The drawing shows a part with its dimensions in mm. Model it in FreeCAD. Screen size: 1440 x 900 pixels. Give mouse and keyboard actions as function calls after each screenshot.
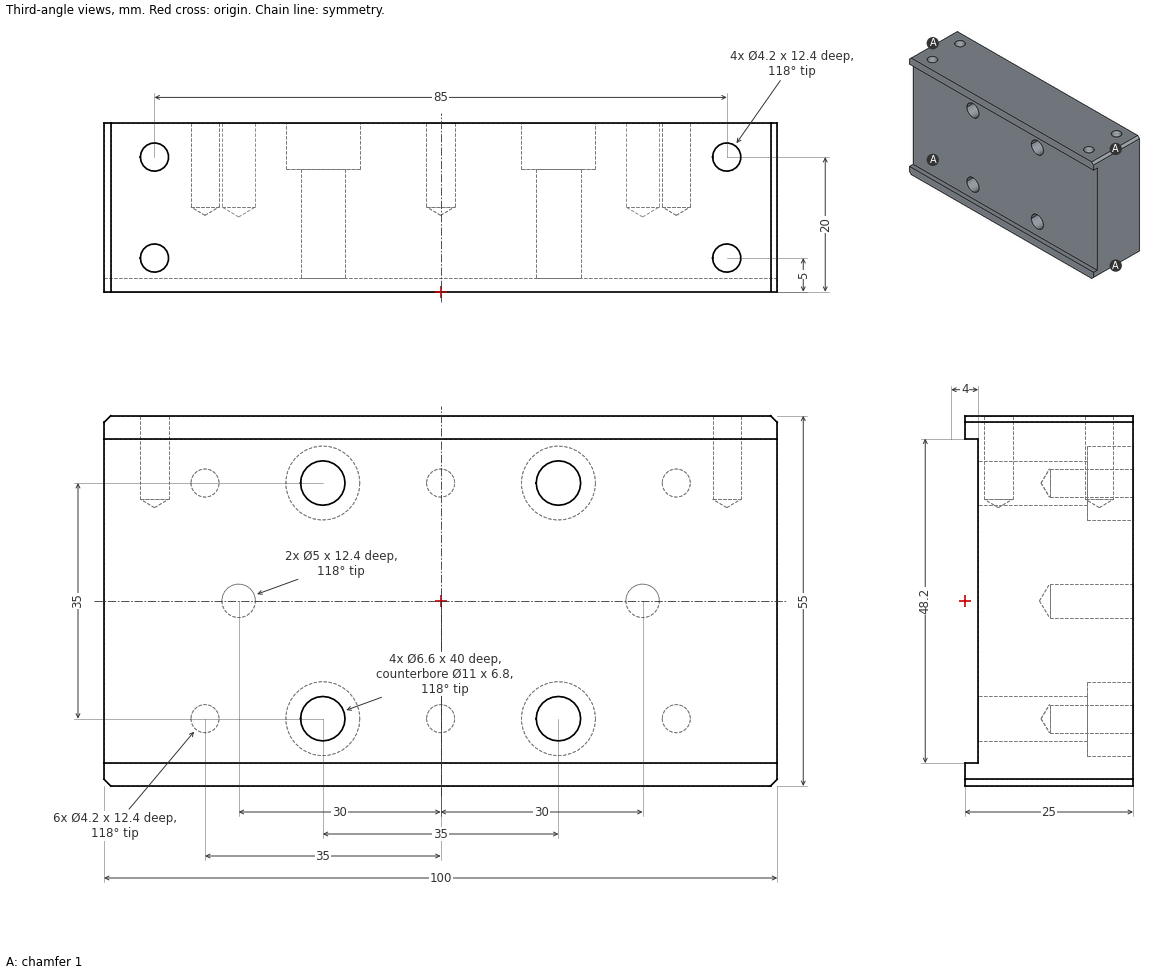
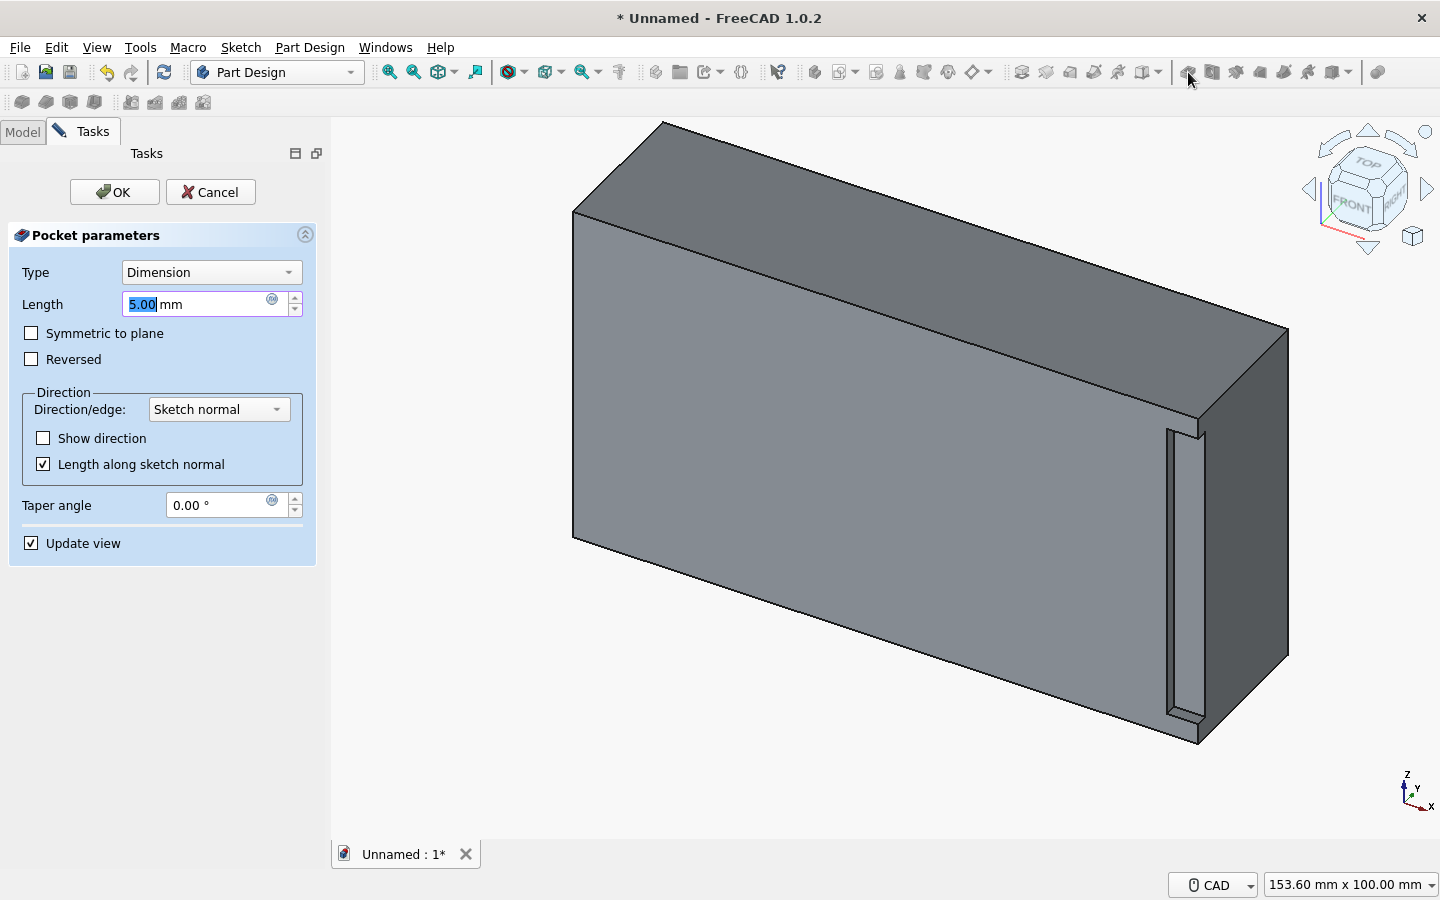
click(212, 272)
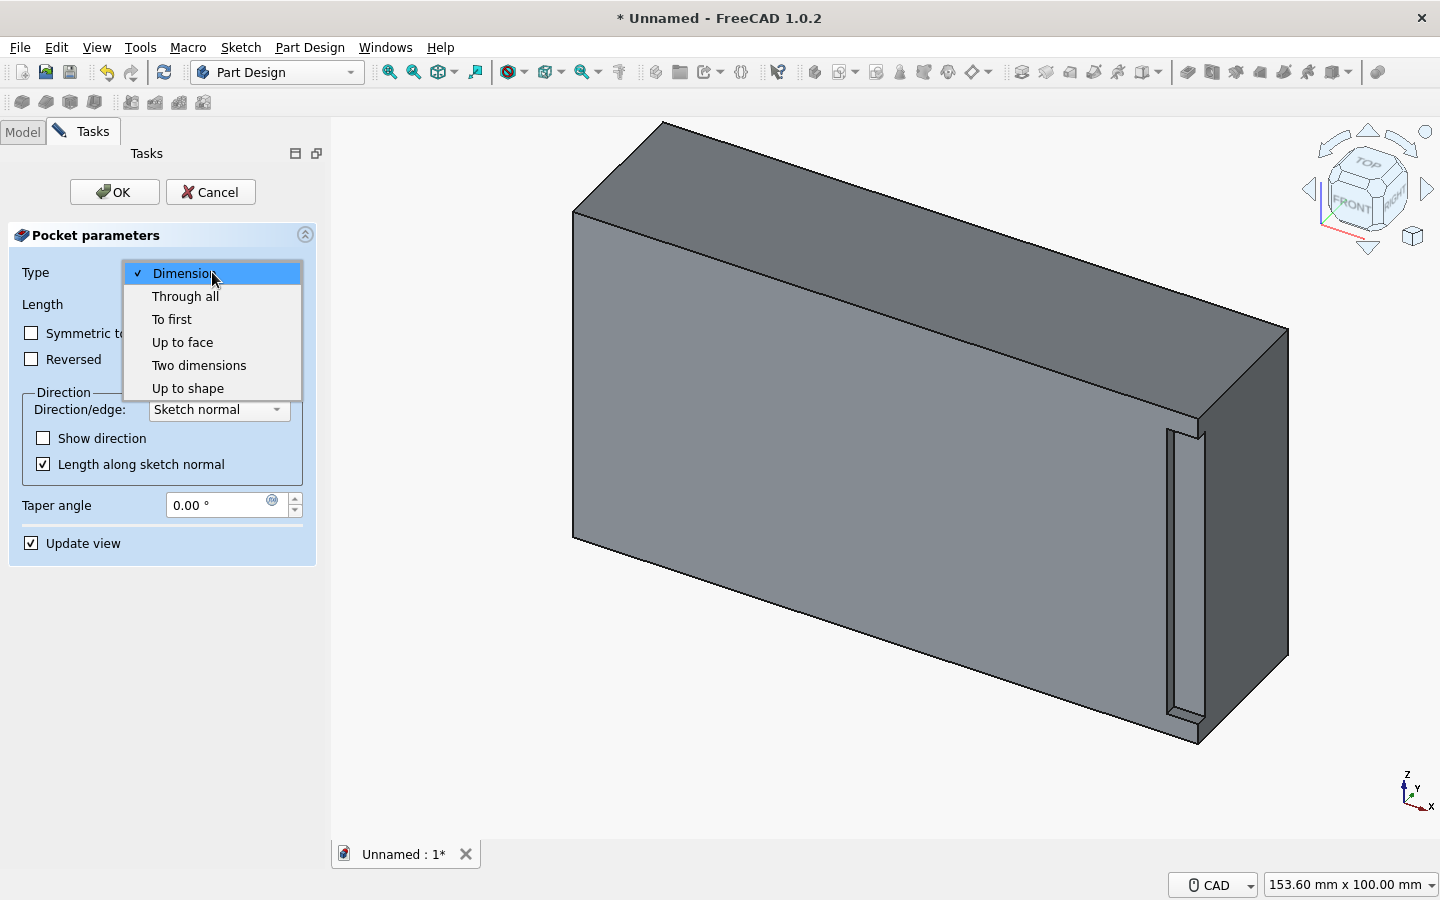
click(212, 296)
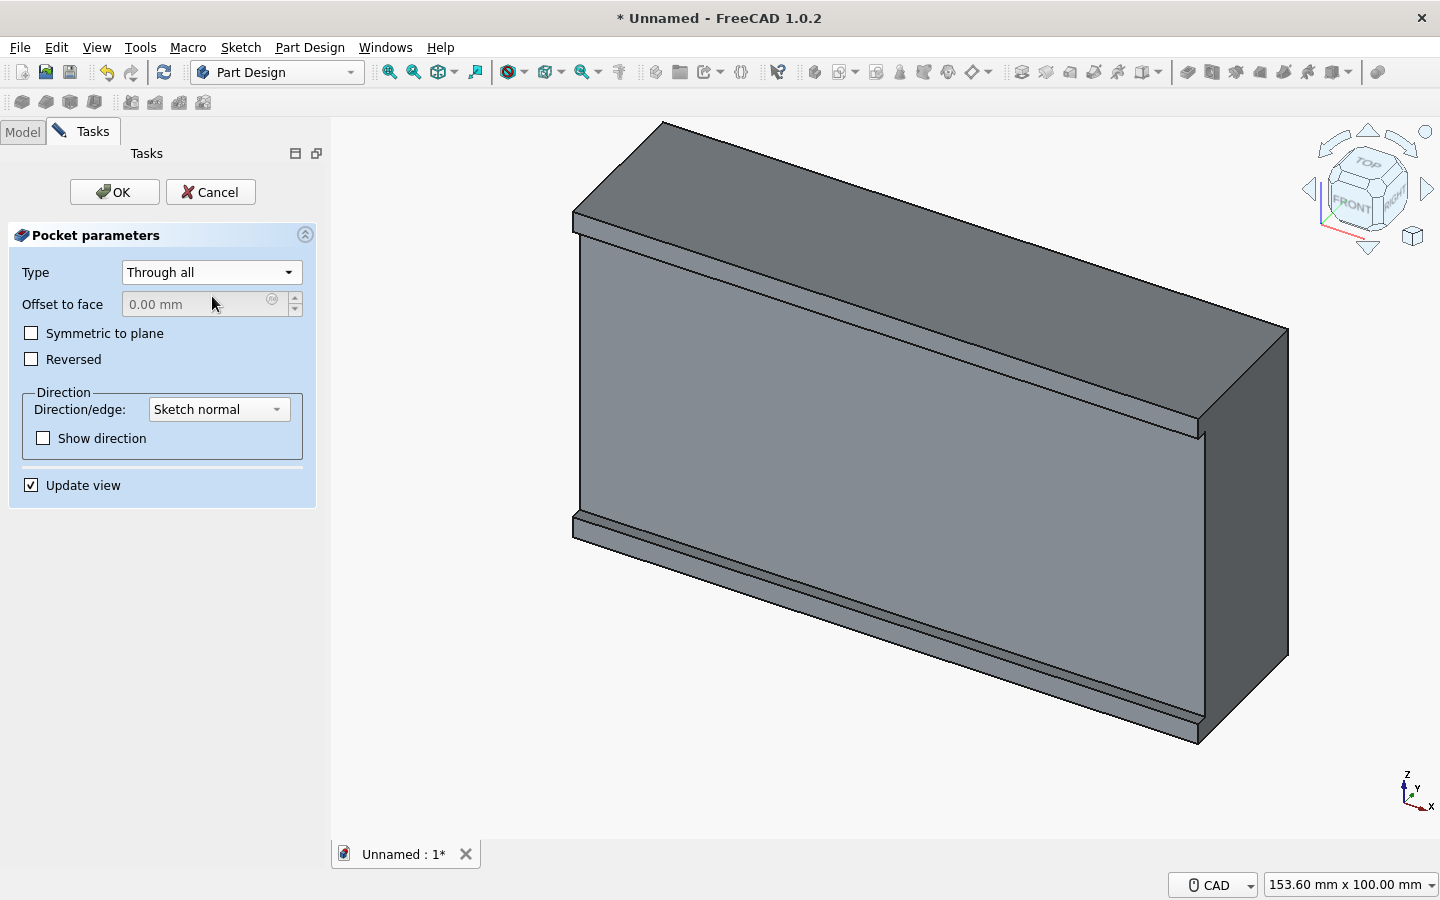
click(115, 192)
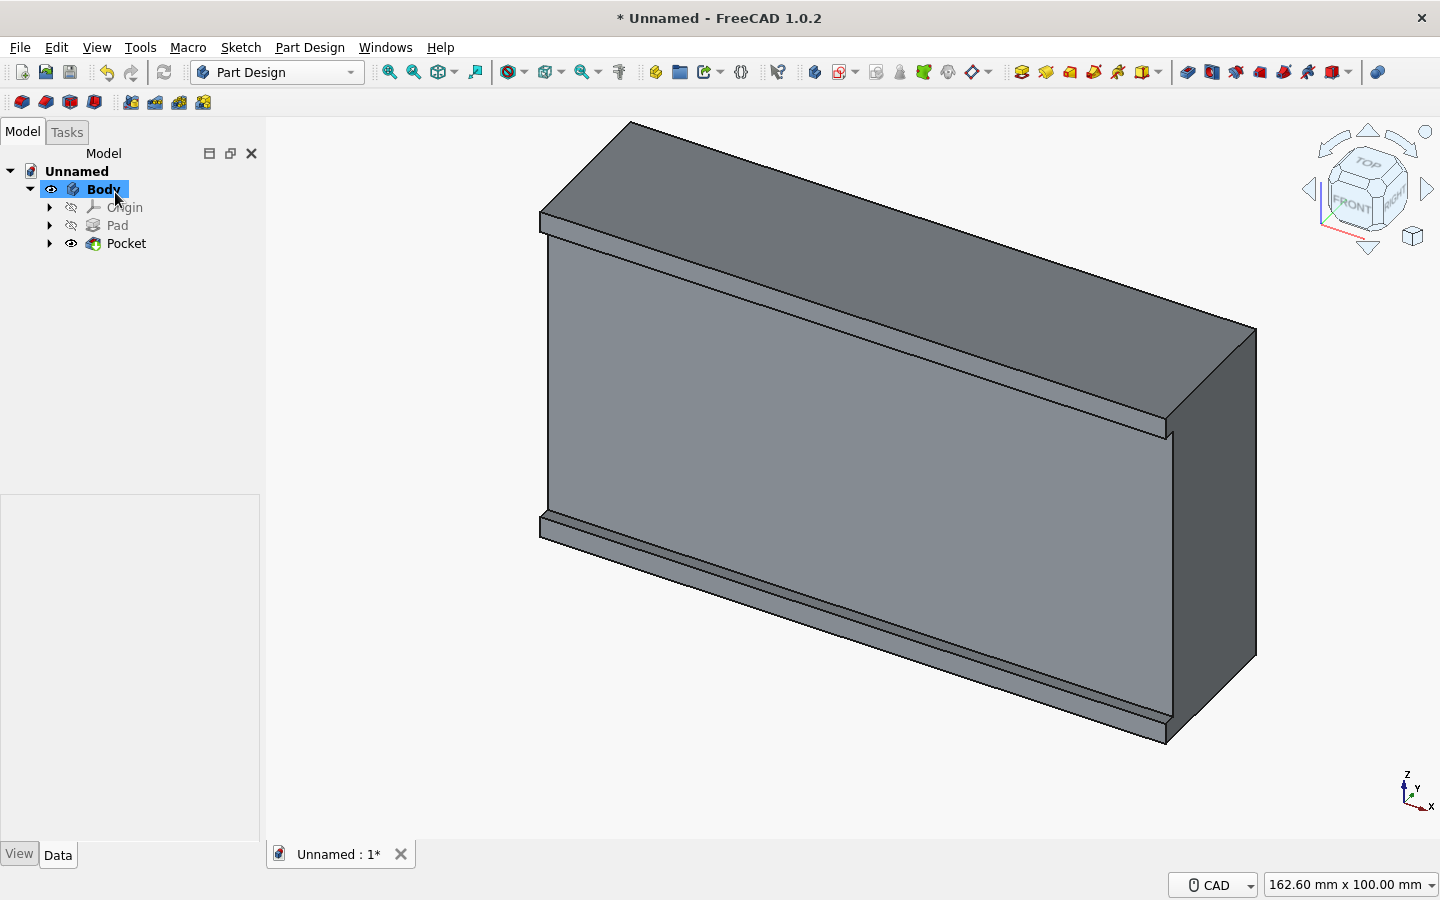
click(1077, 329)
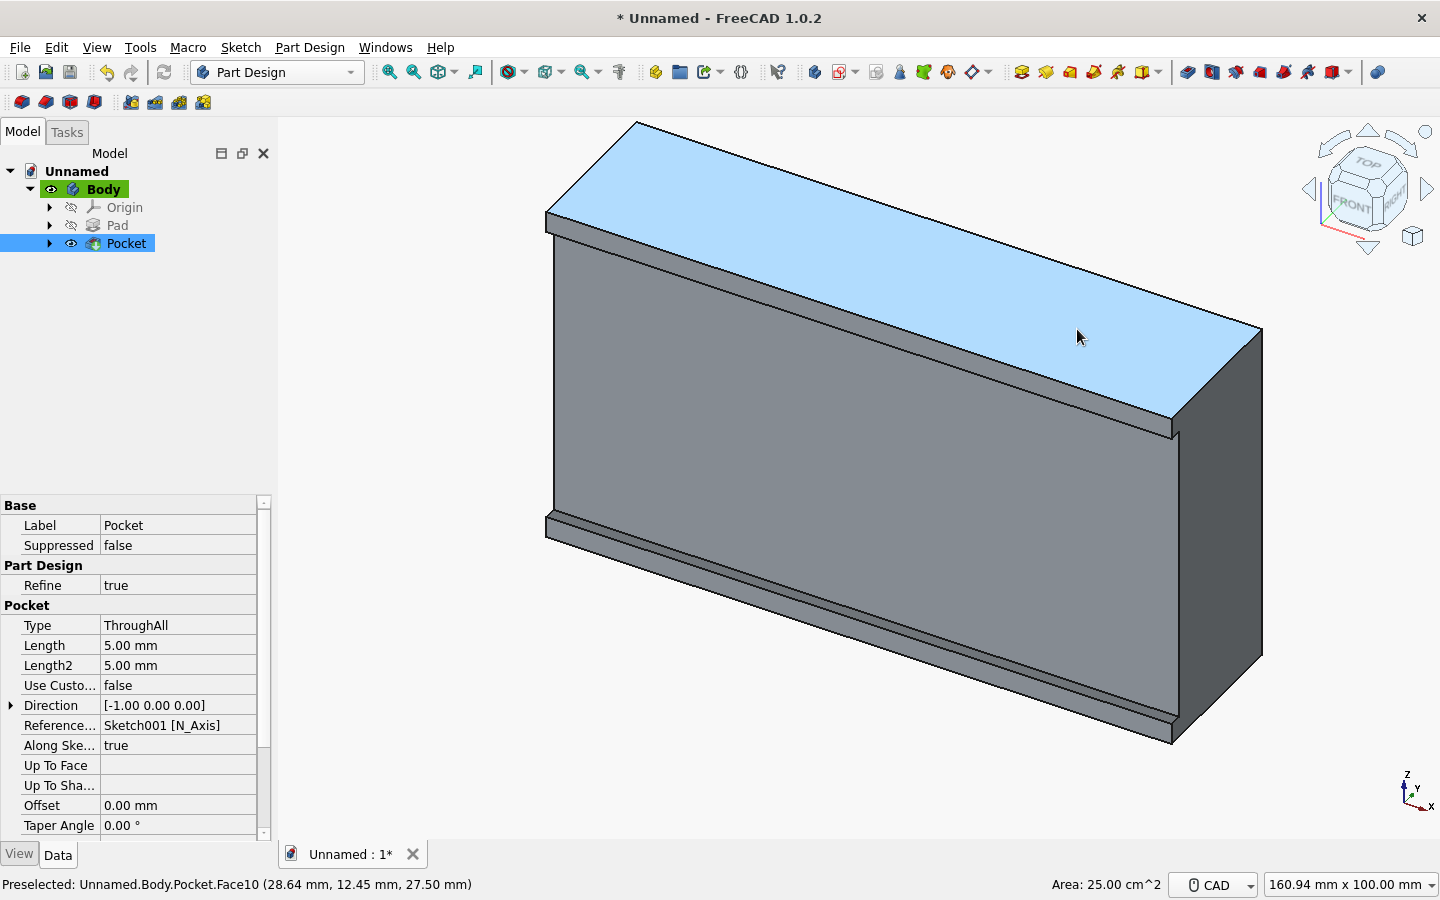
click(840, 72)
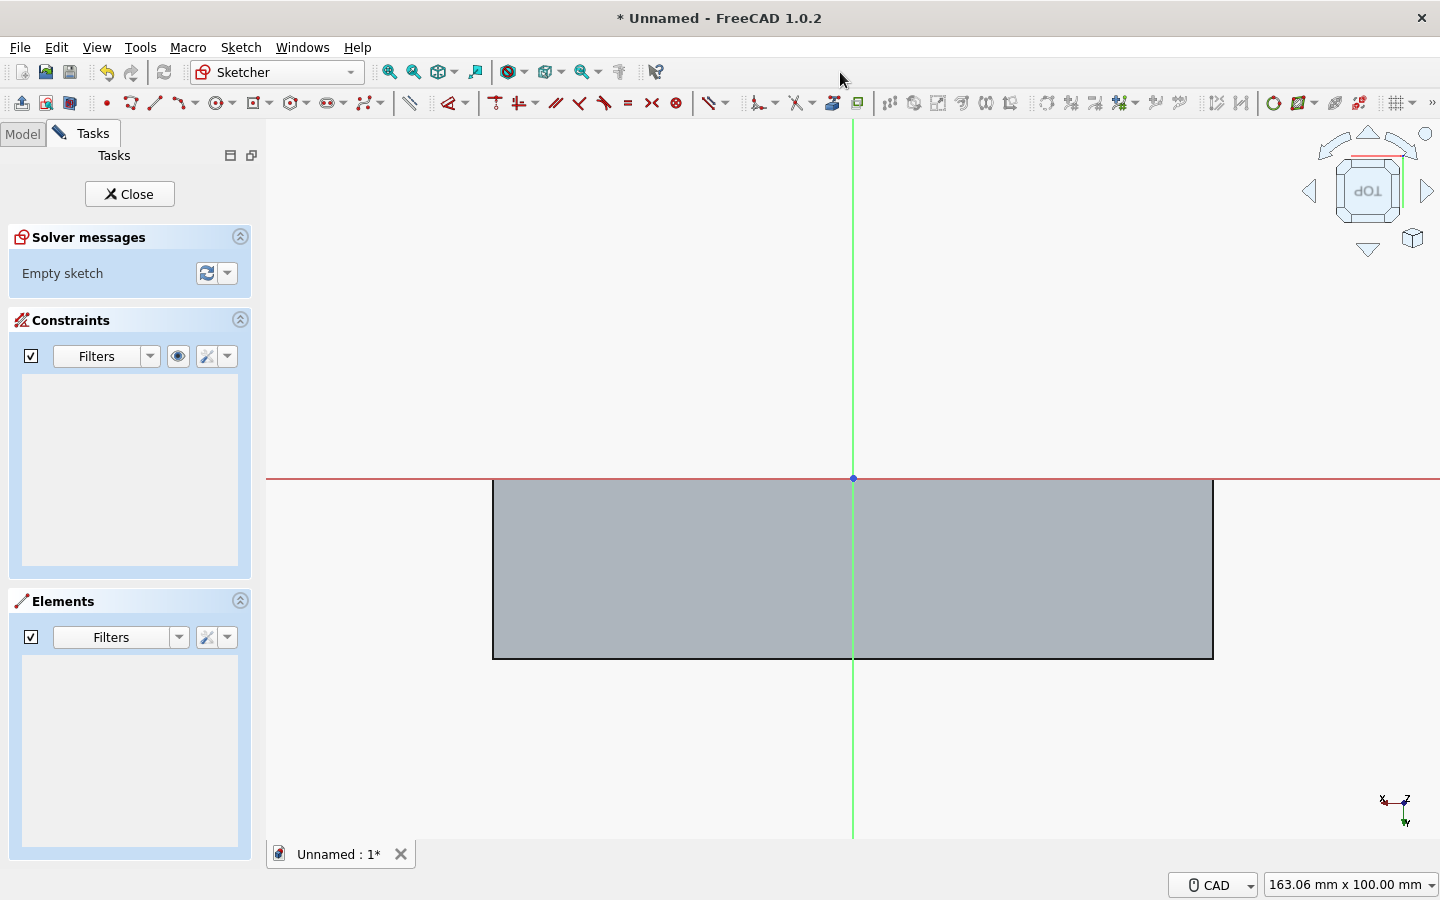
click(216, 104)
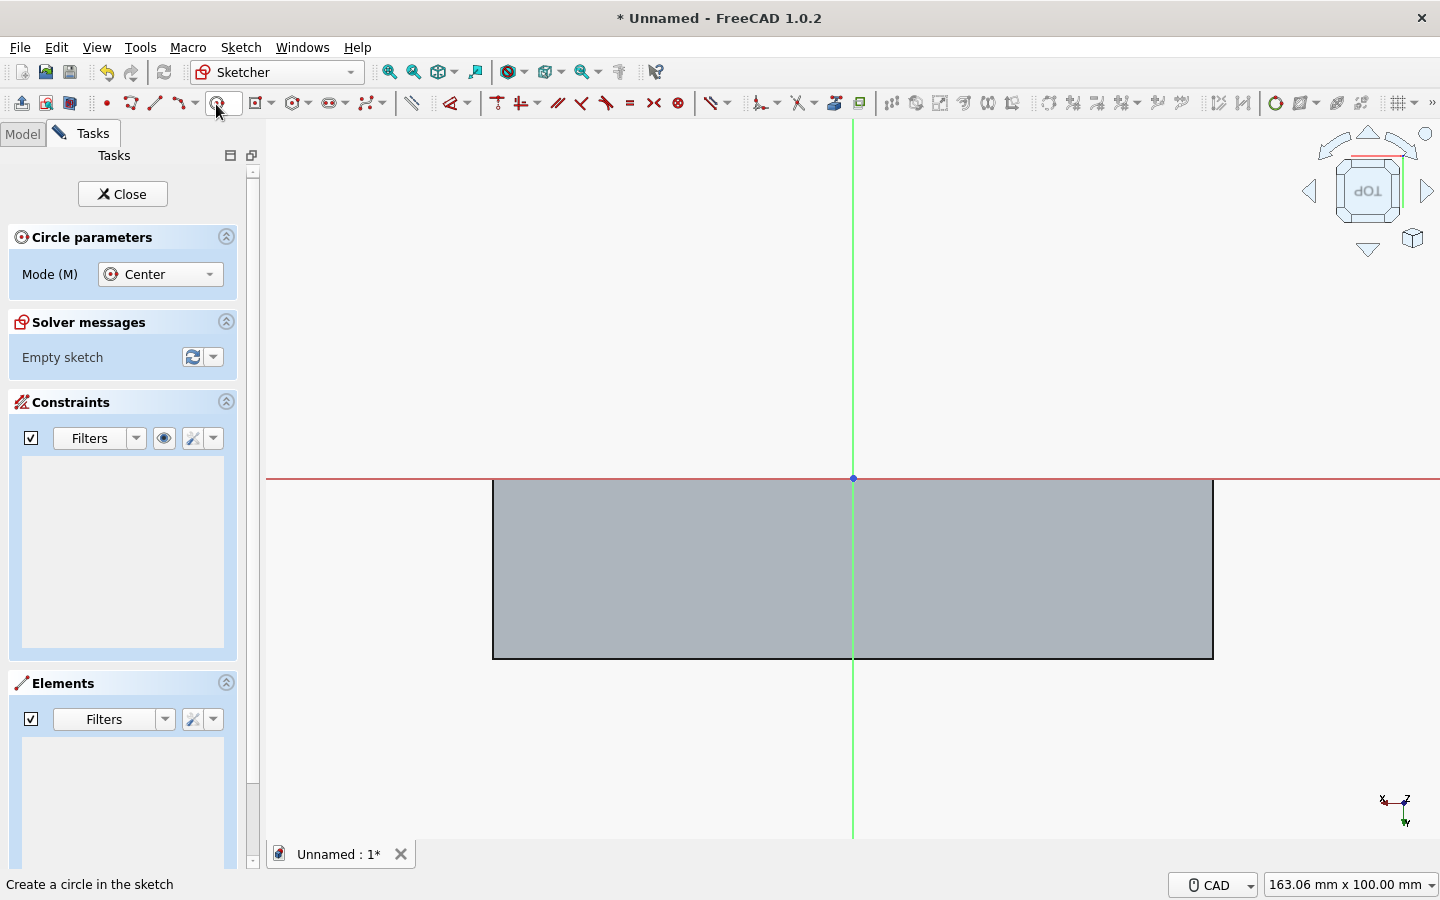
scroll(547, 623, up, 3)